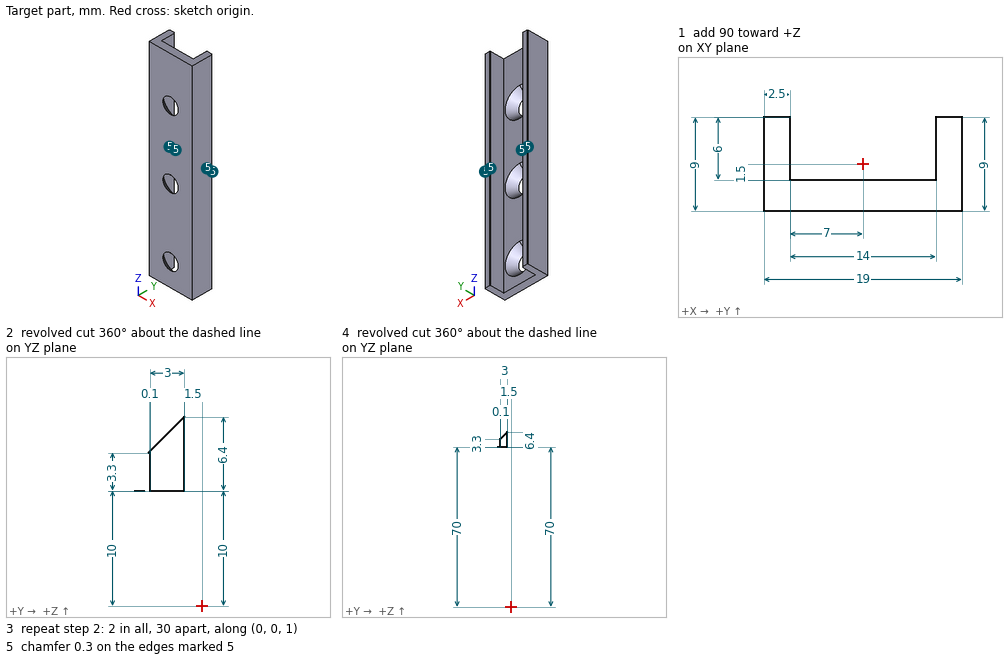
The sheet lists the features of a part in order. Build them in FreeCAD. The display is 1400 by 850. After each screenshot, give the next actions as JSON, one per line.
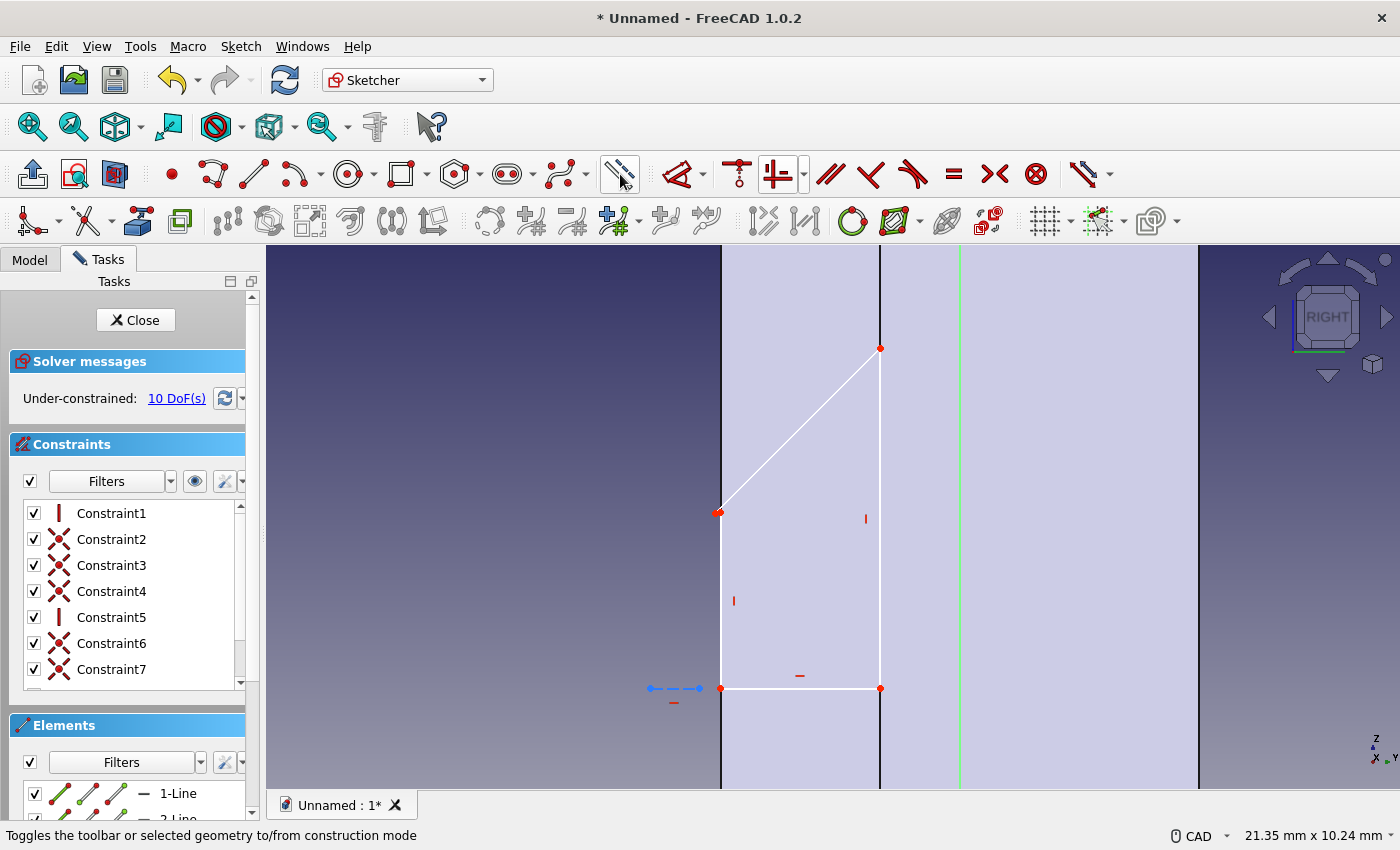
{"action": "scroll", "coordinate": [719, 513], "scroll_direction": "up", "scroll_amount": 10}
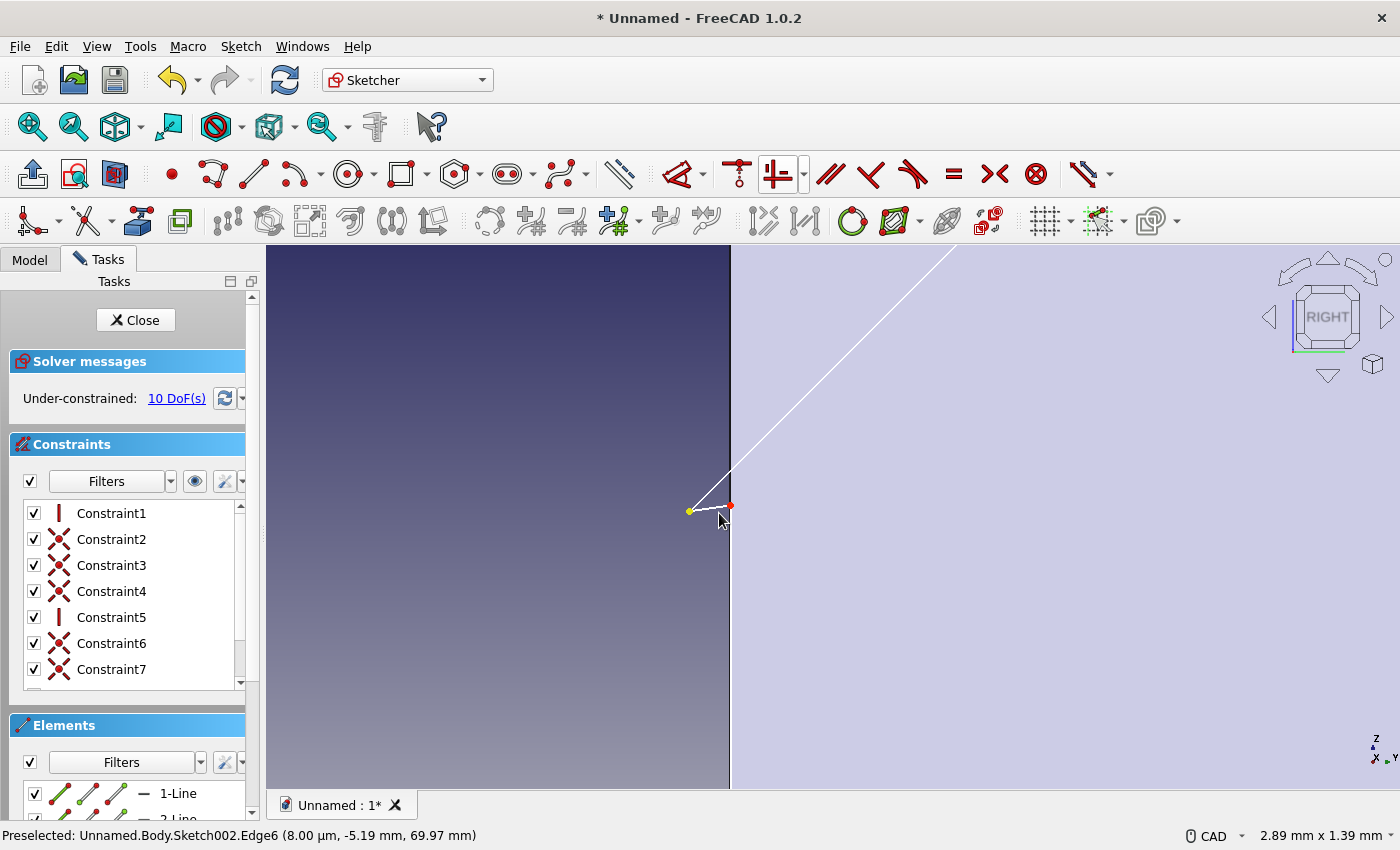
{"action": "left_click", "coordinate": [714, 508]}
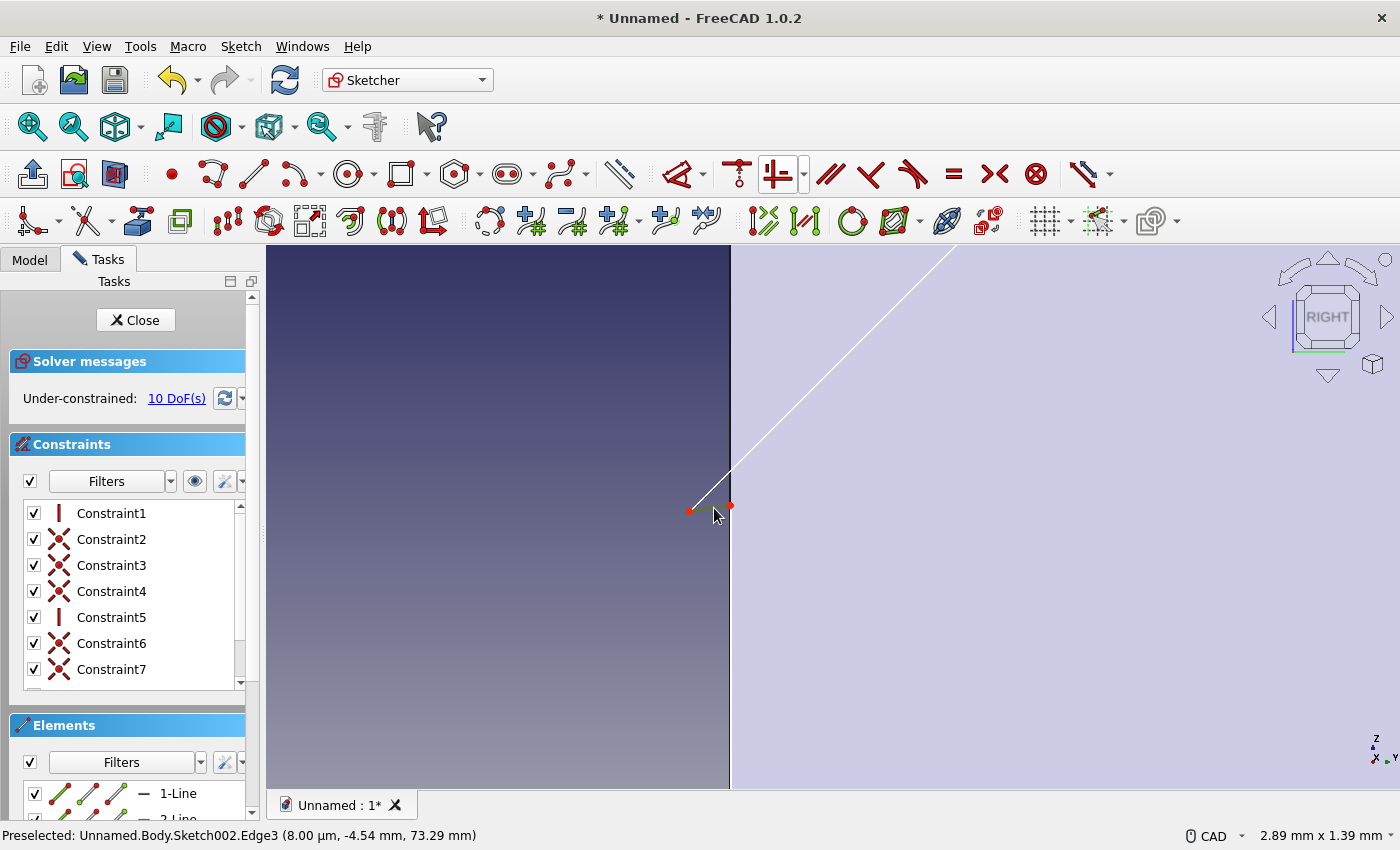
{"action": "key", "text": "h"}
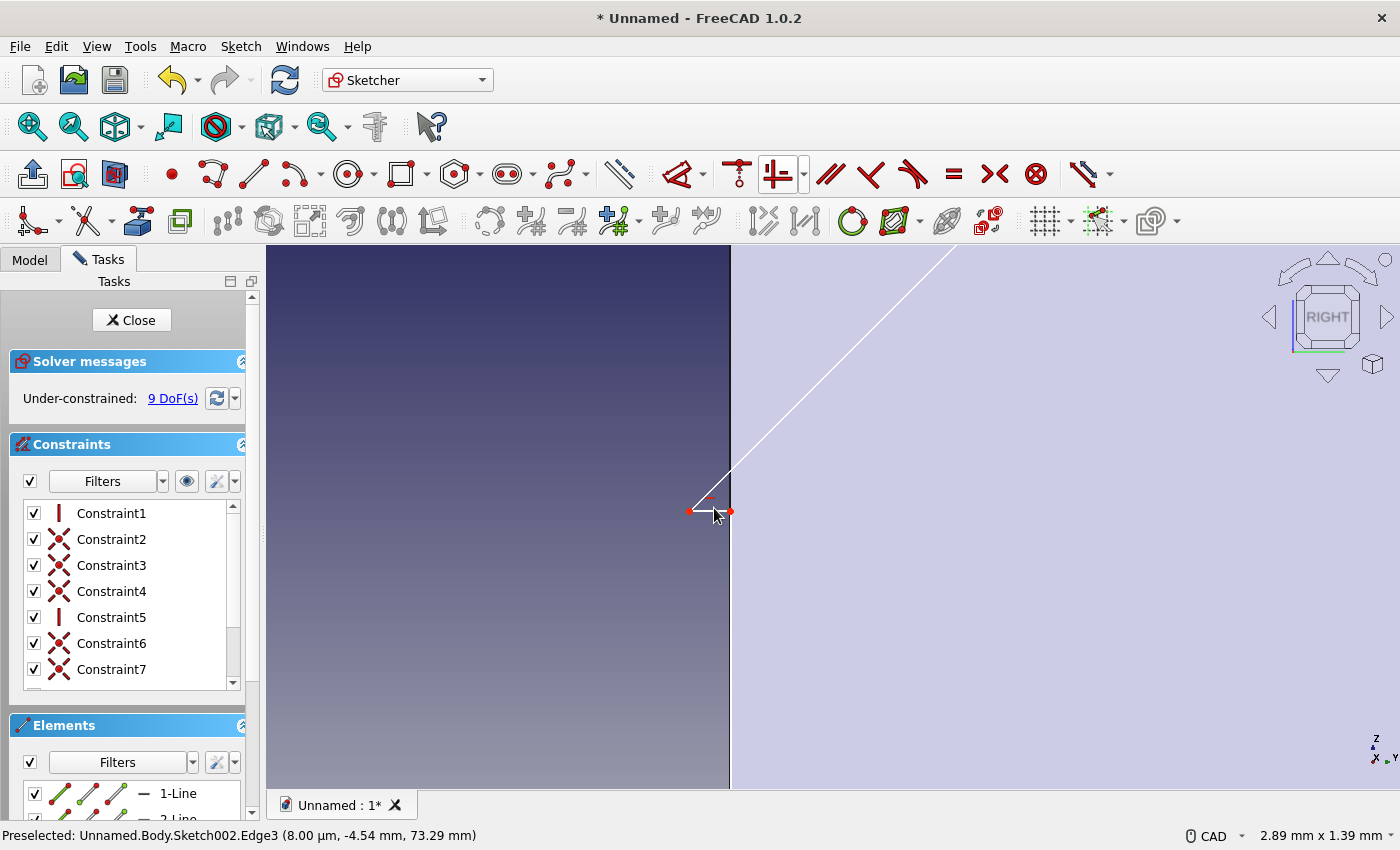
{"action": "left_click", "coordinate": [676, 174]}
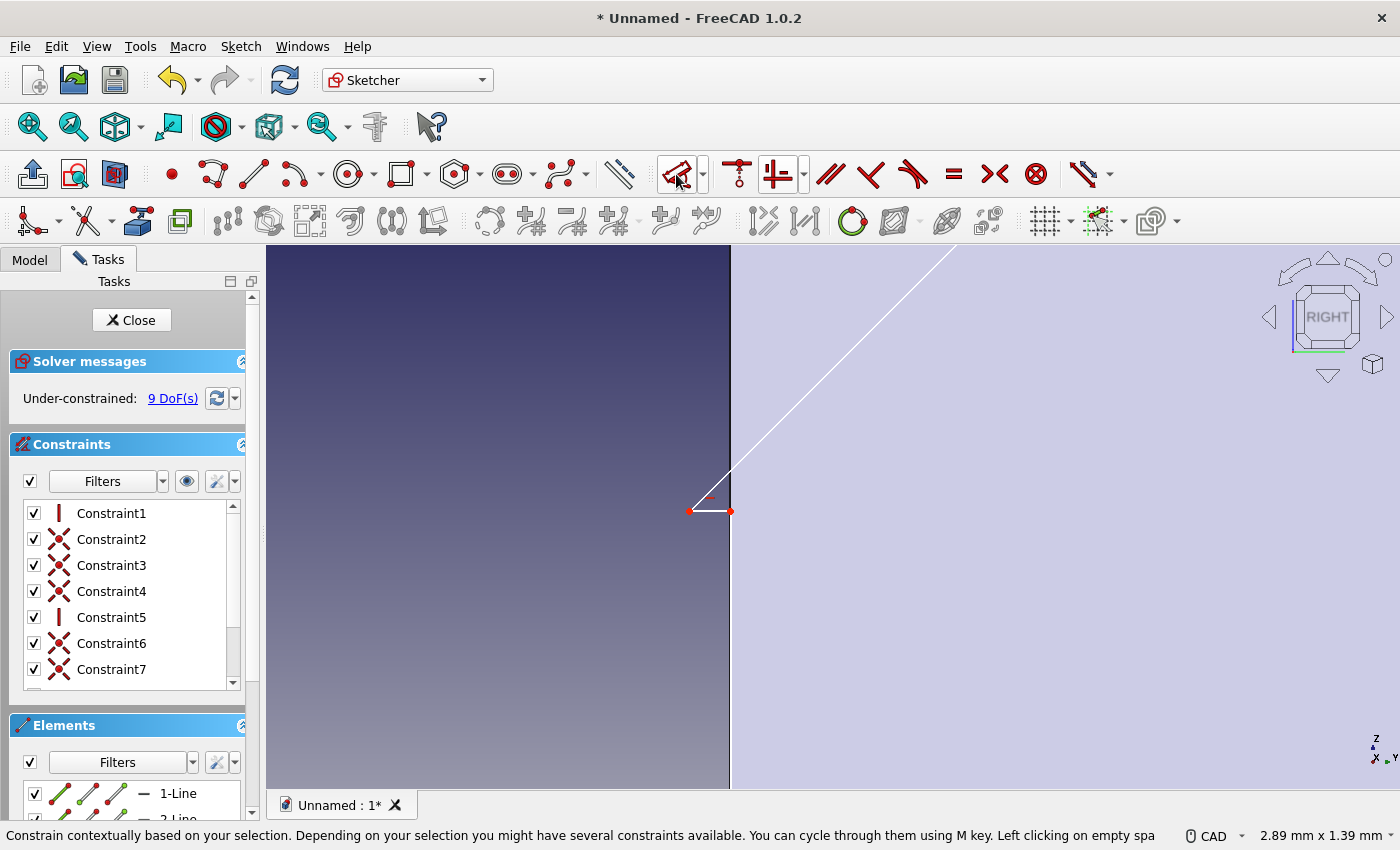
{"action": "scroll", "coordinate": [719, 513], "scroll_direction": "down", "scroll_amount": 10}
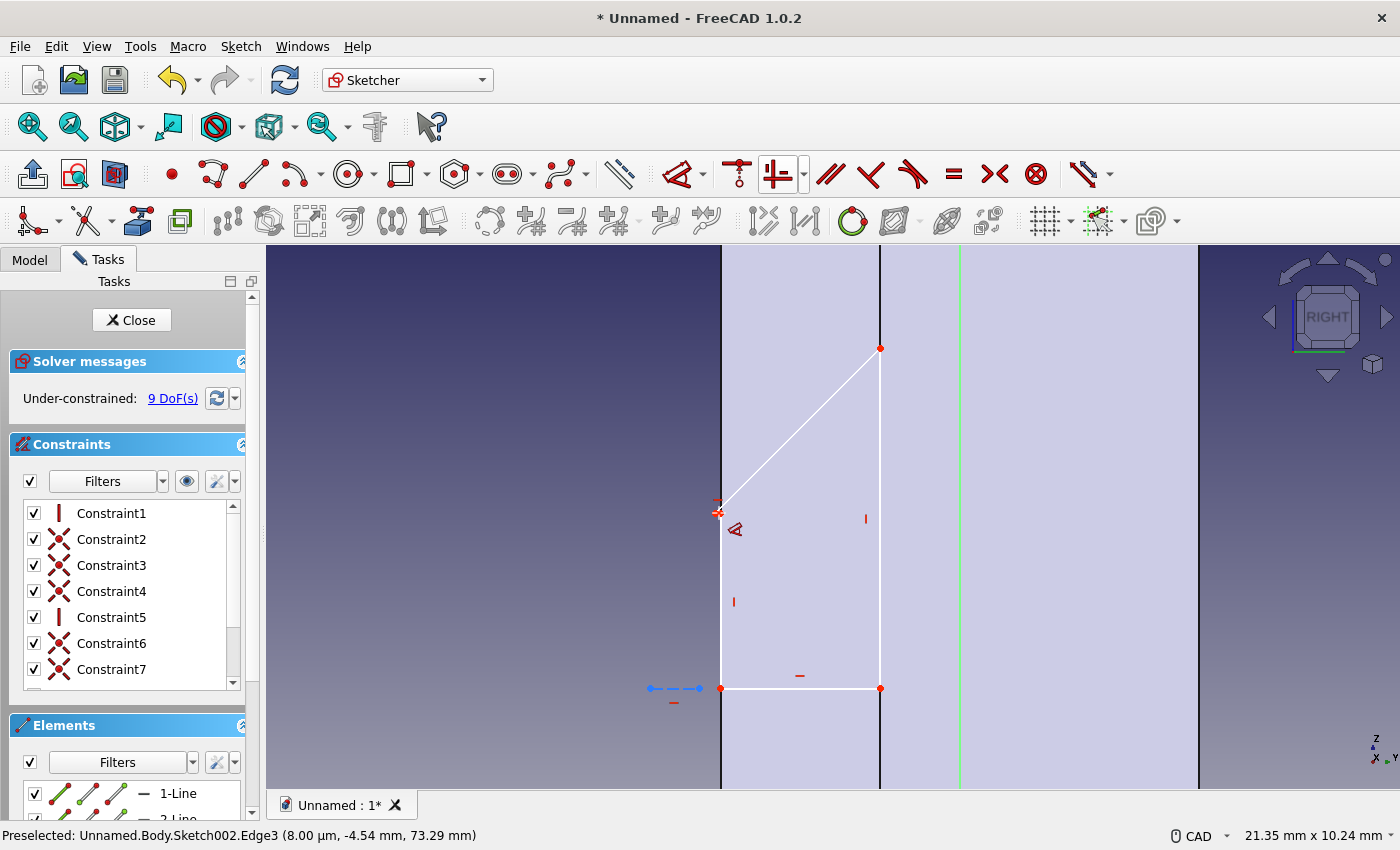
{"action": "left_click", "coordinate": [769, 689]}
{"action": "left_click", "coordinate": [801, 723]}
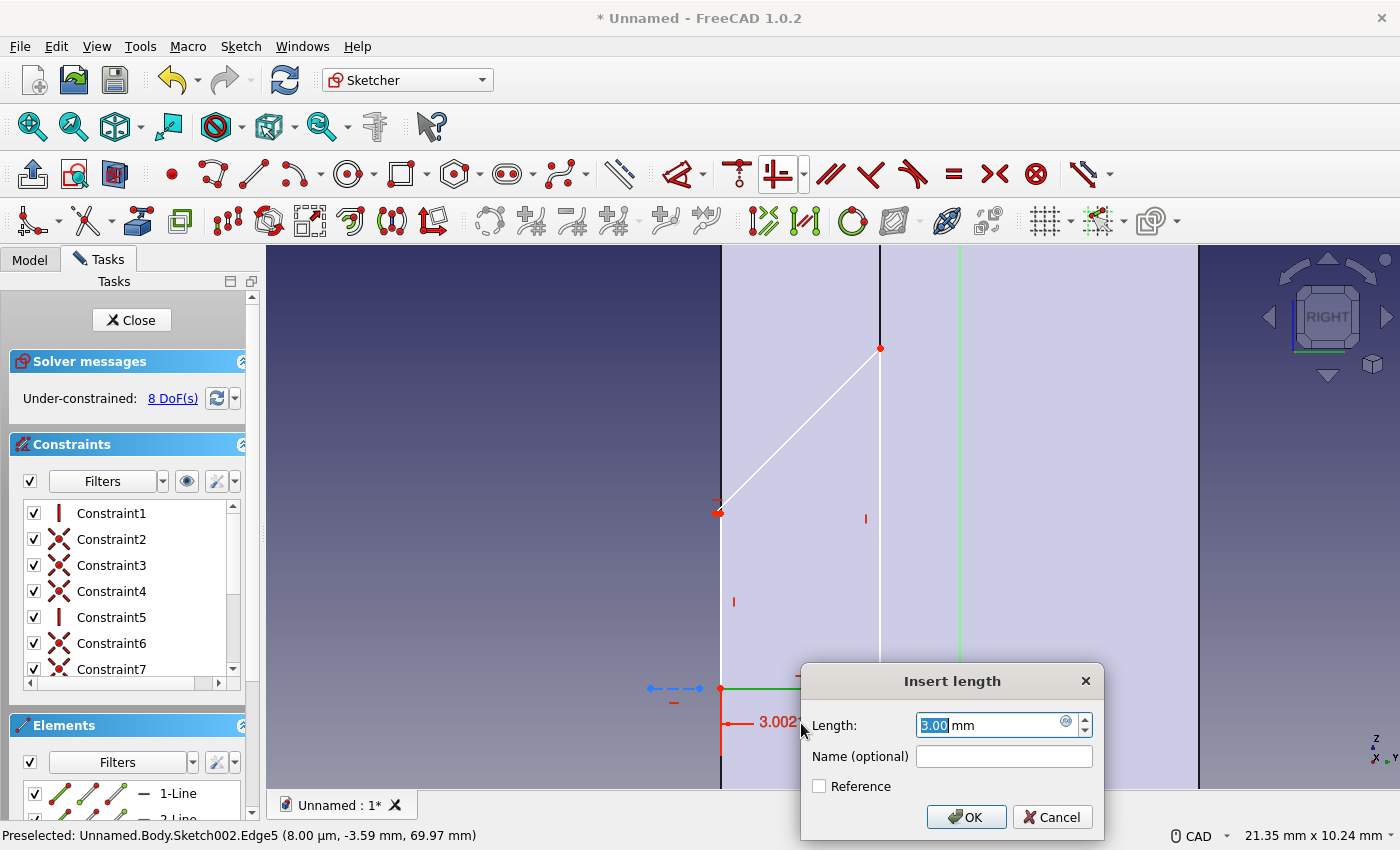
{"action": "type", "text": "3"}
{"action": "key", "text": "Return"}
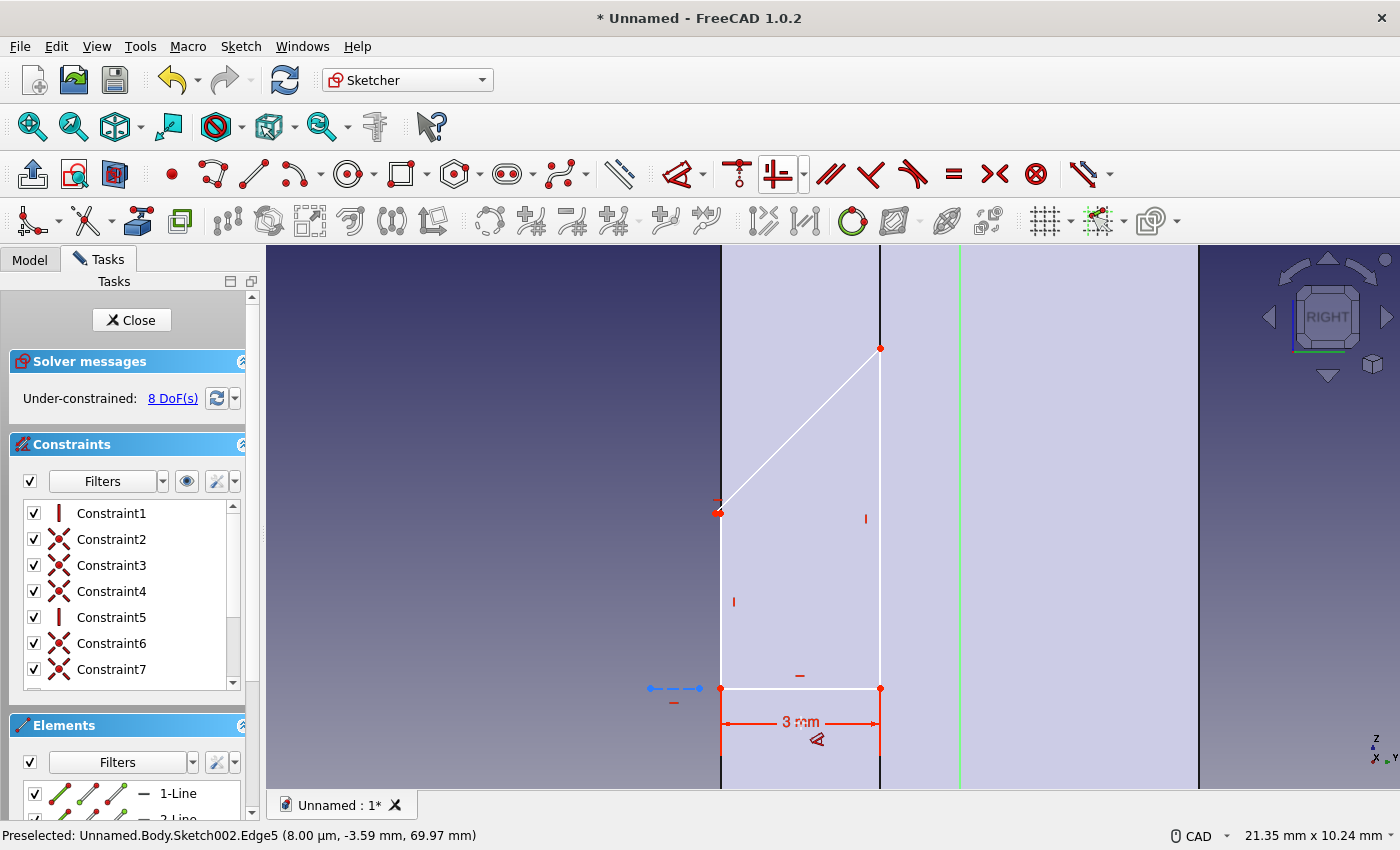
{"action": "left_click", "coordinate": [880, 587]}
{"action": "left_click", "coordinate": [914, 519]}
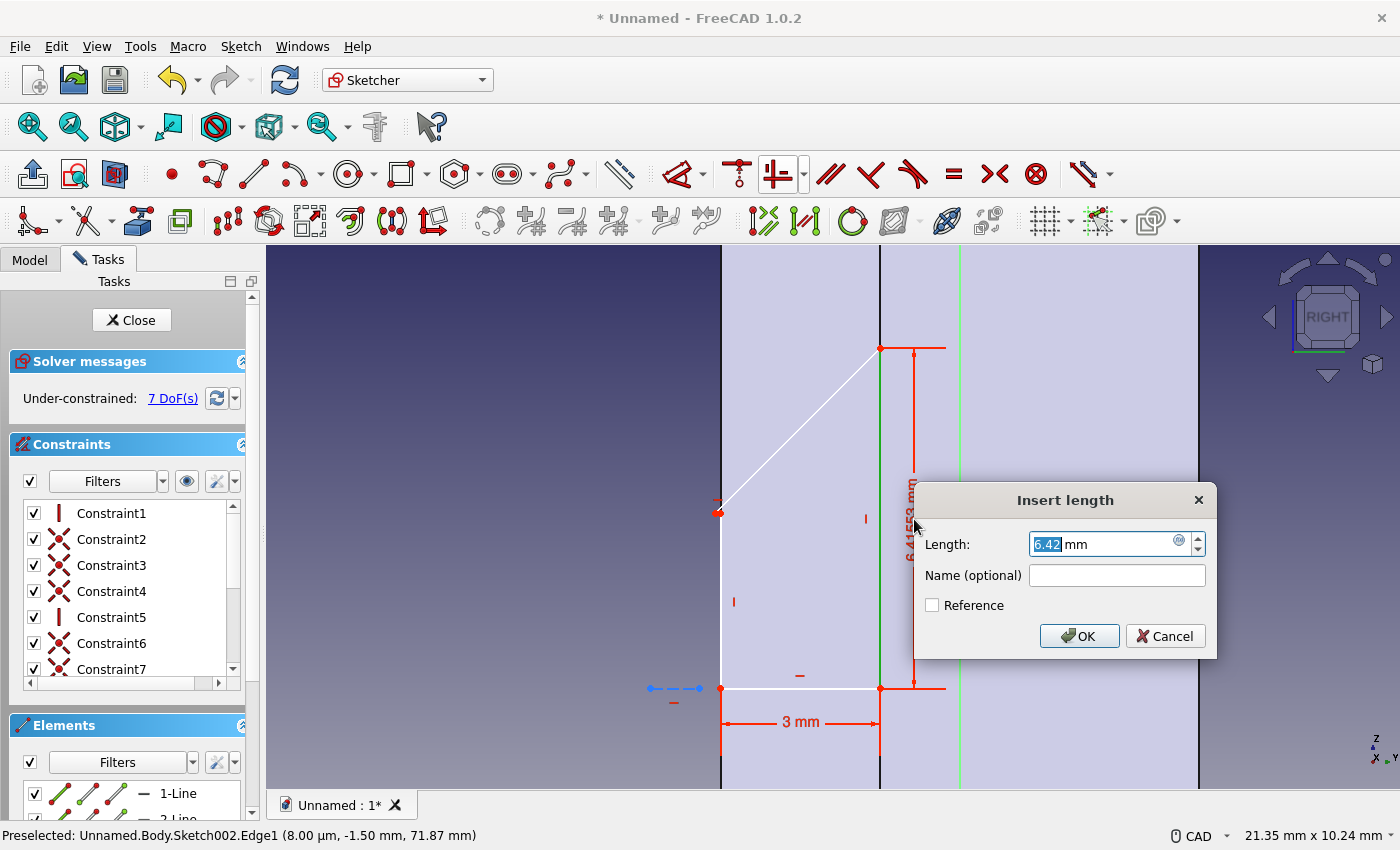
{"action": "type", "text": "6.4"}
{"action": "key", "text": "Return"}